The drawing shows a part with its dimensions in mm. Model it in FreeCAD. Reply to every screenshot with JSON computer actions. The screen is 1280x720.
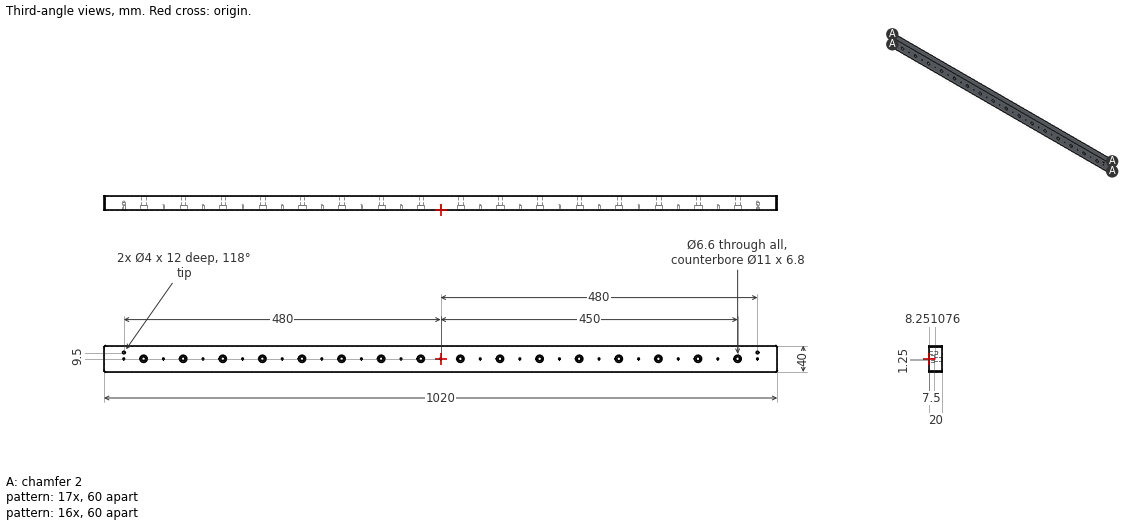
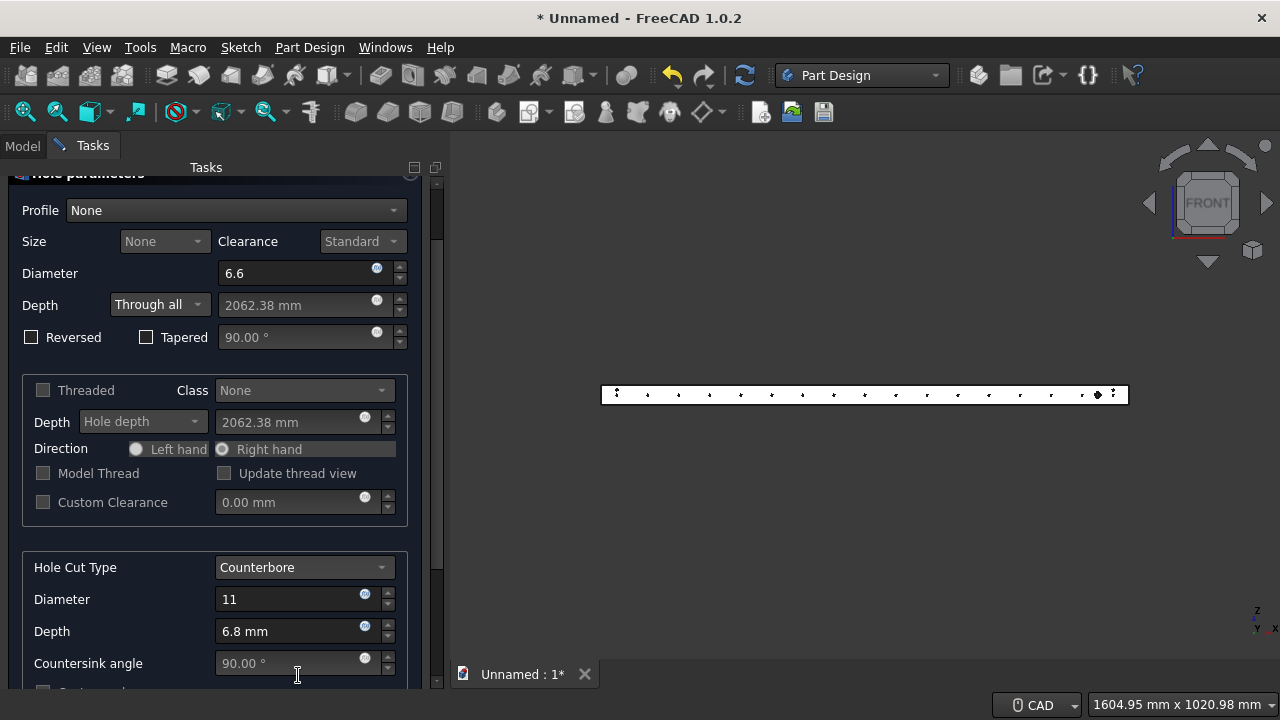
{"action": "scroll", "coordinate": [437, 432], "scroll_direction": "up", "scroll_amount": 3}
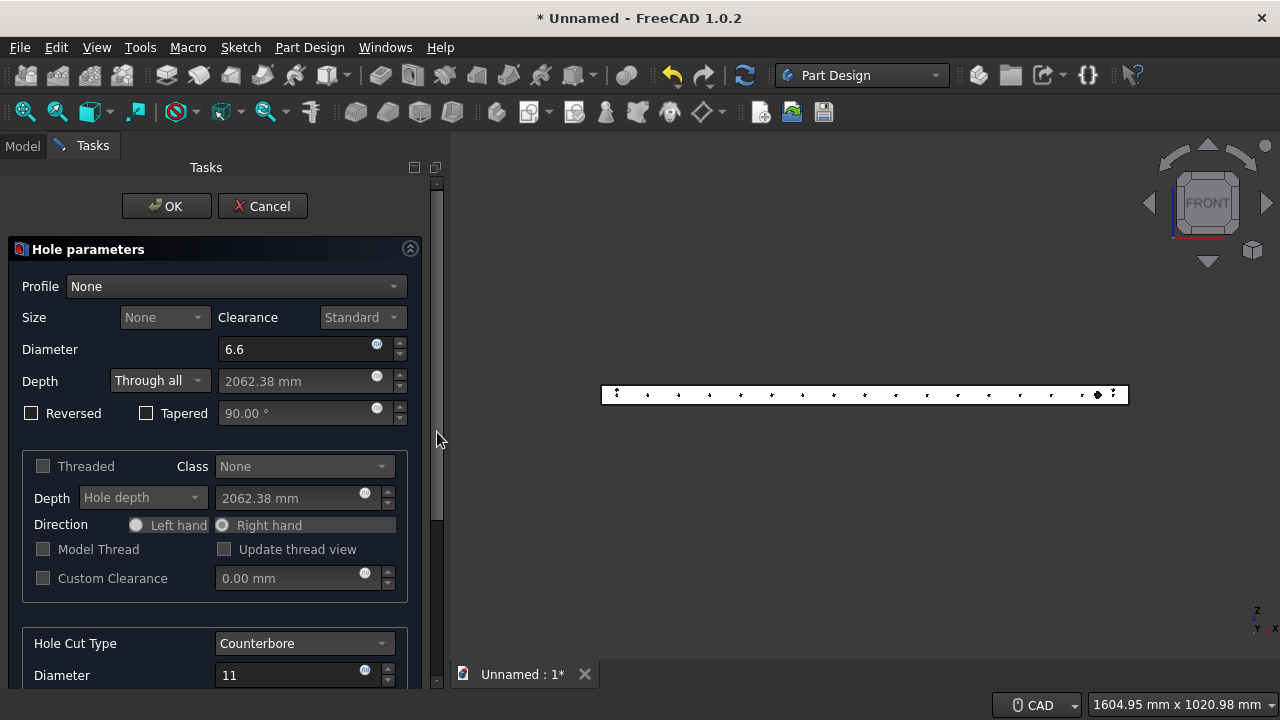
{"action": "left_click", "coordinate": [167, 206]}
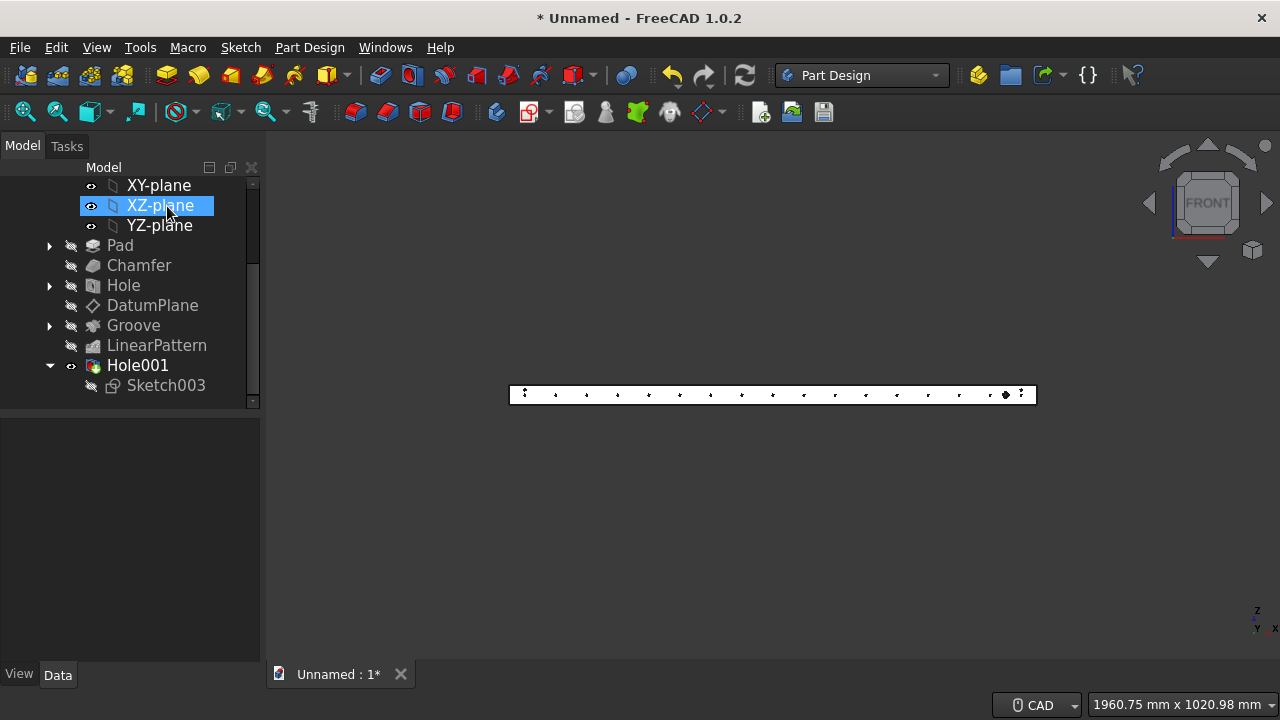
{"action": "left_click", "coordinate": [116, 366]}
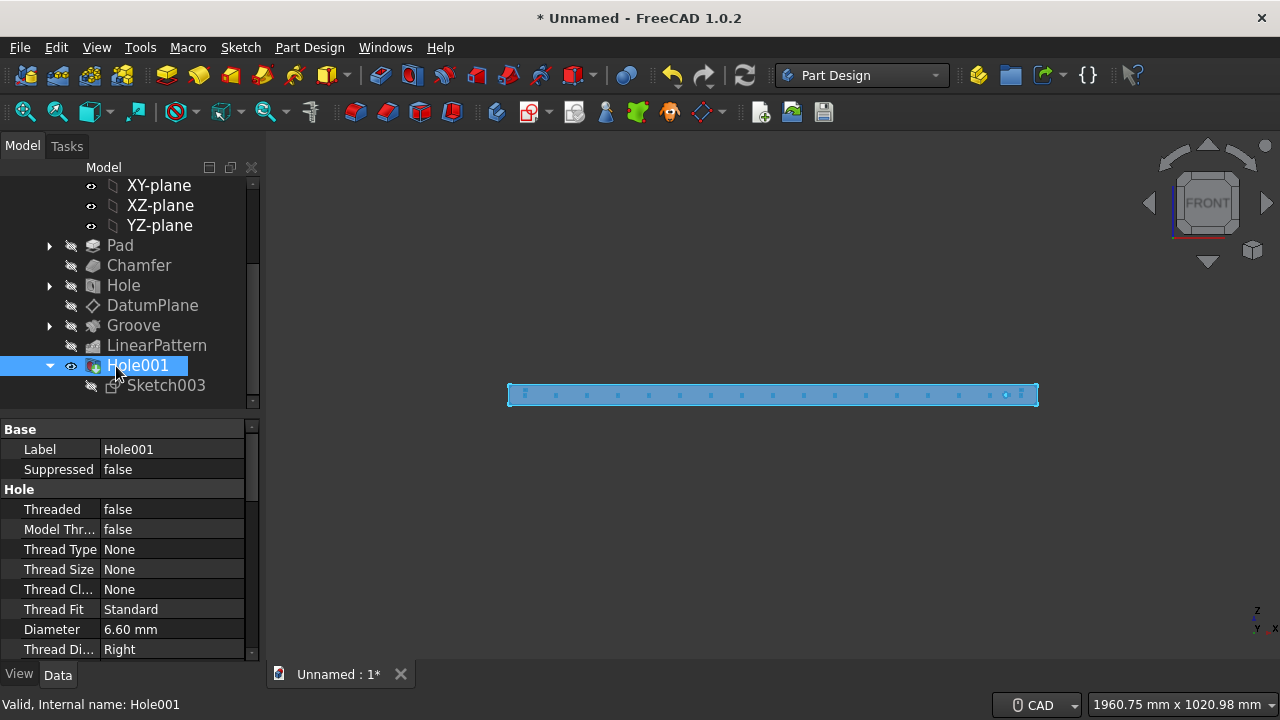
{"action": "left_click", "coordinate": [58, 76]}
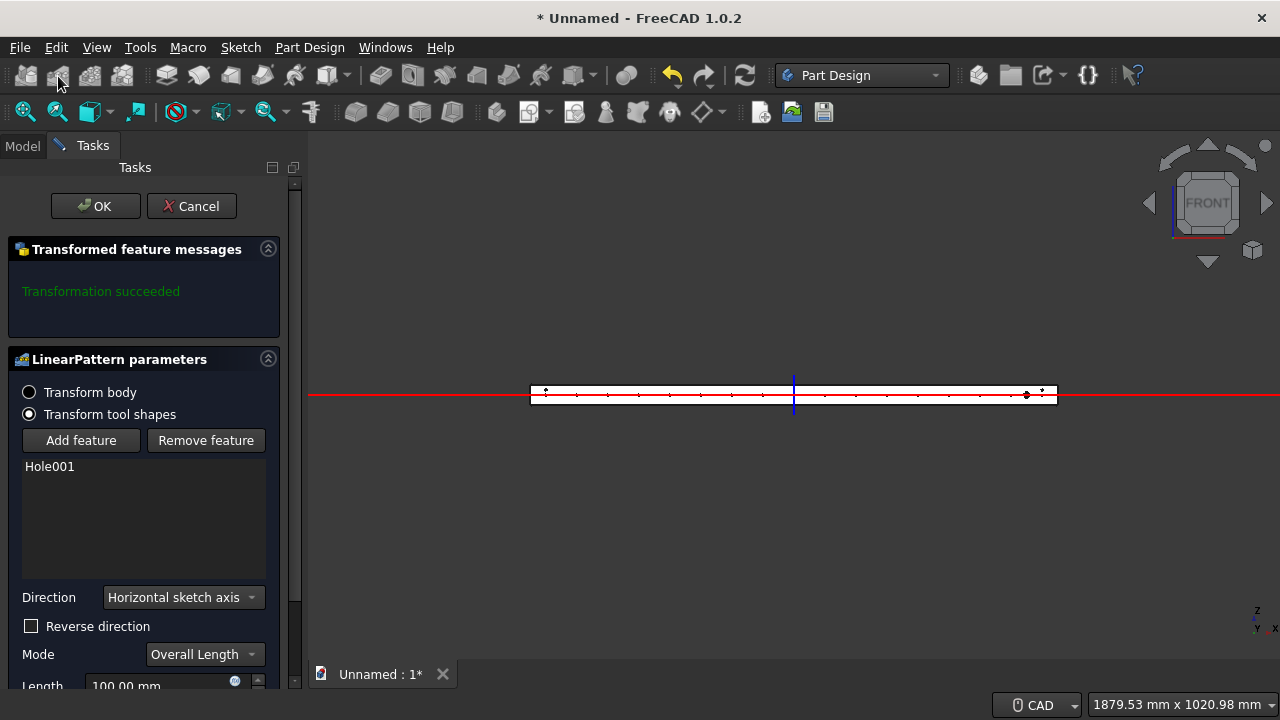
{"action": "left_click", "coordinate": [184, 598]}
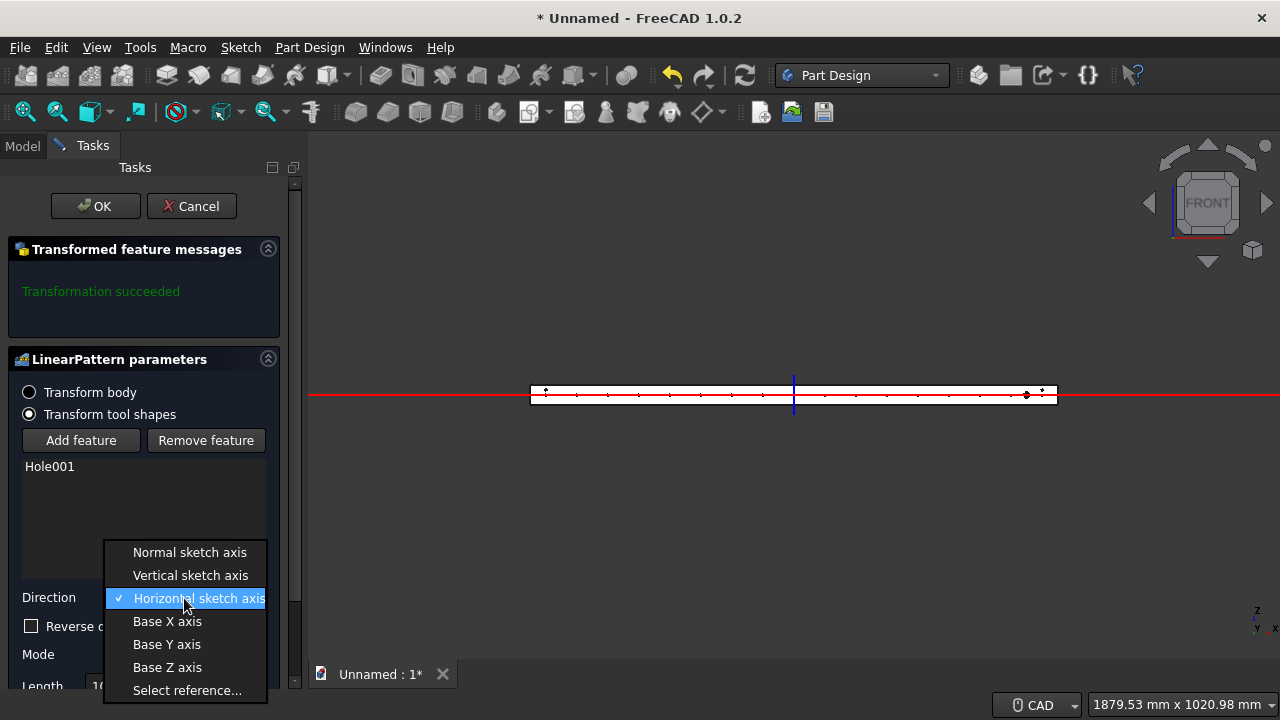
{"action": "left_click", "coordinate": [184, 622]}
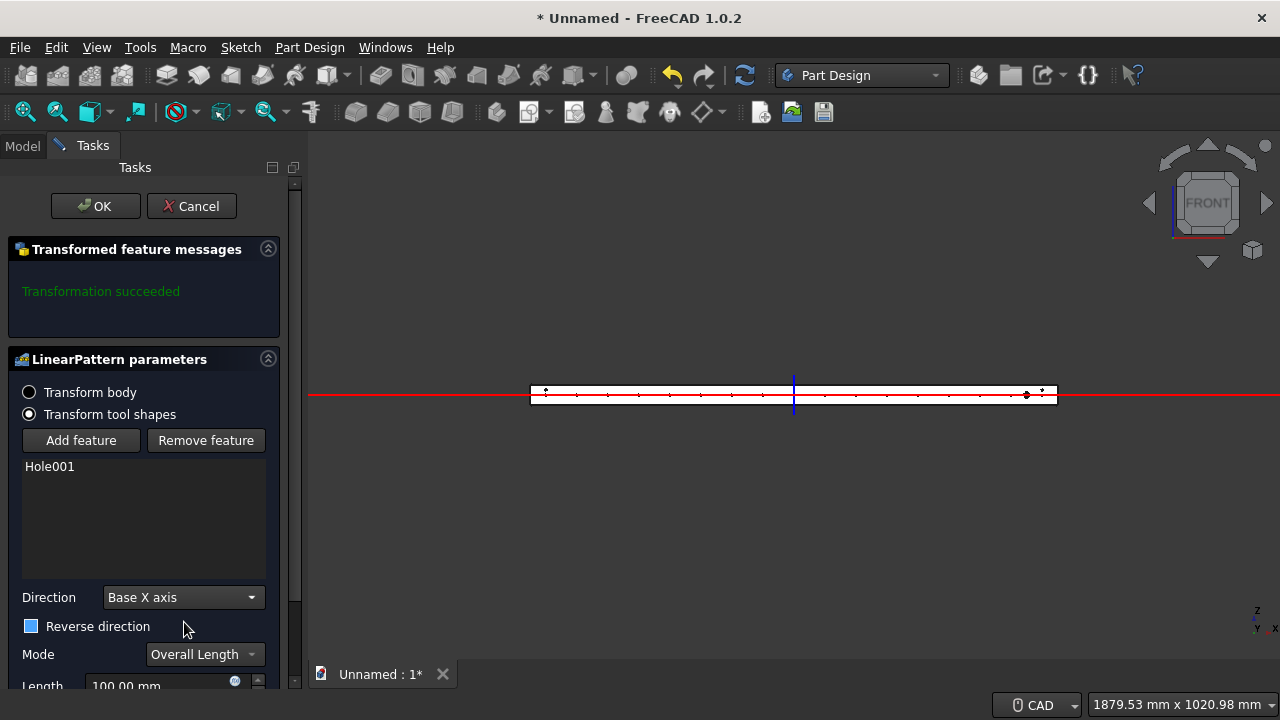
{"action": "left_click", "coordinate": [206, 654]}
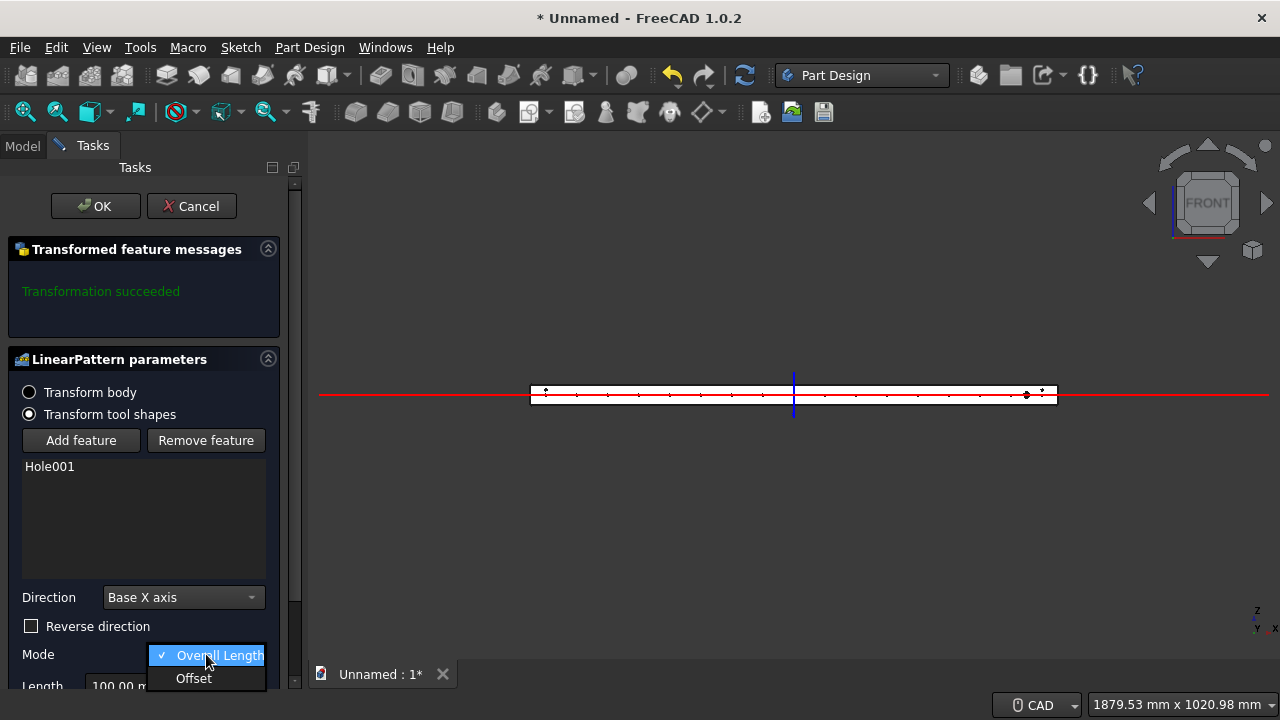
{"action": "left_click", "coordinate": [206, 678]}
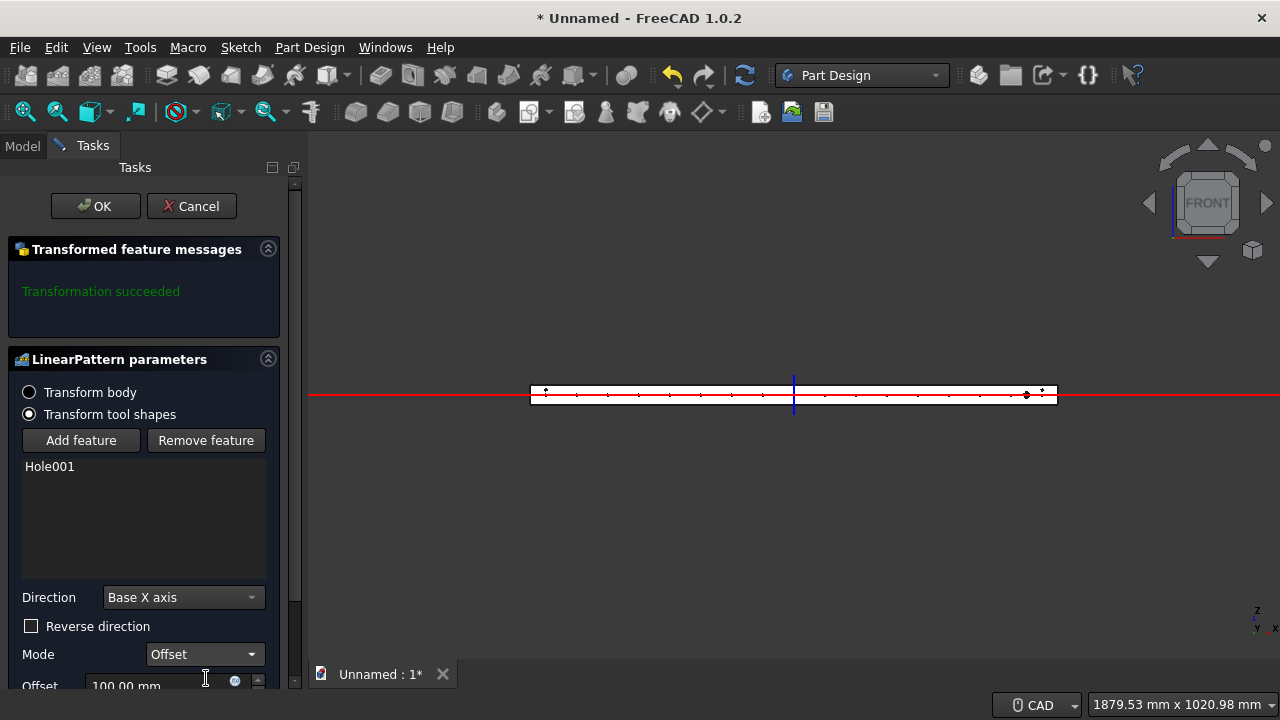
{"action": "scroll", "coordinate": [295, 432], "scroll_direction": "down", "scroll_amount": 2}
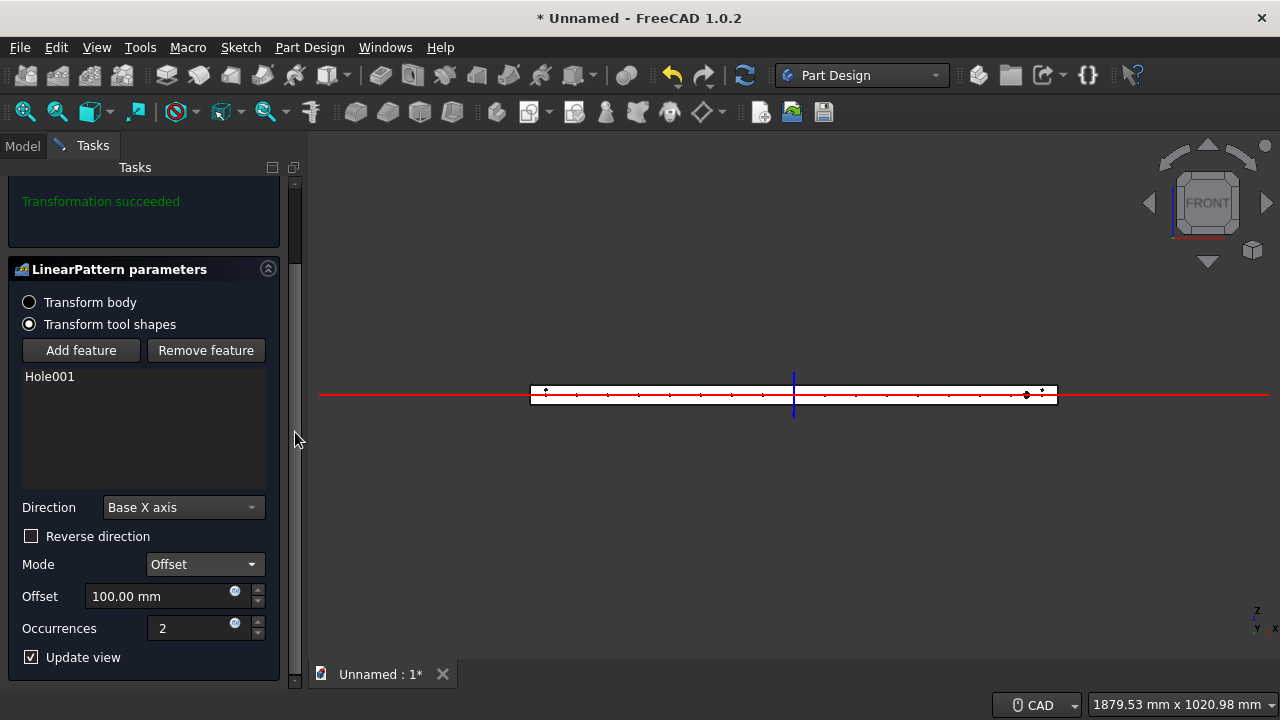
{"action": "triple_click", "coordinate": [168, 596]}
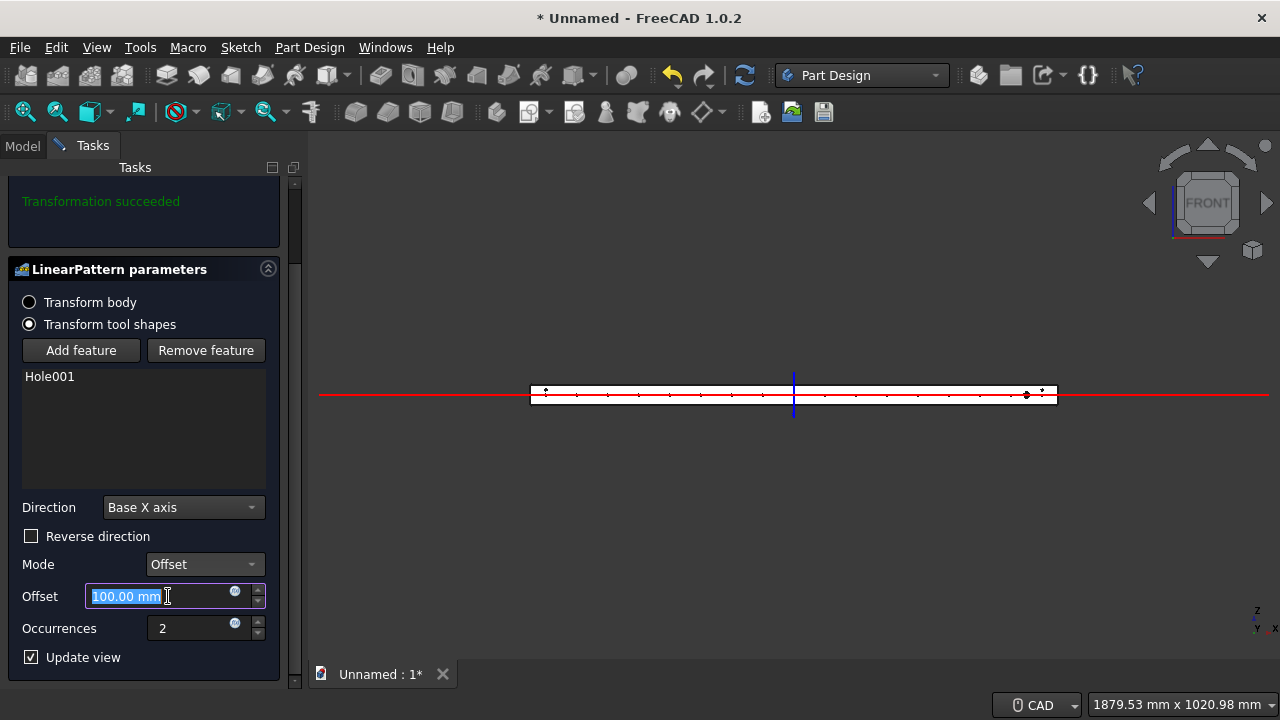
{"action": "type", "text": "60"}
{"action": "key", "text": "Tab"}